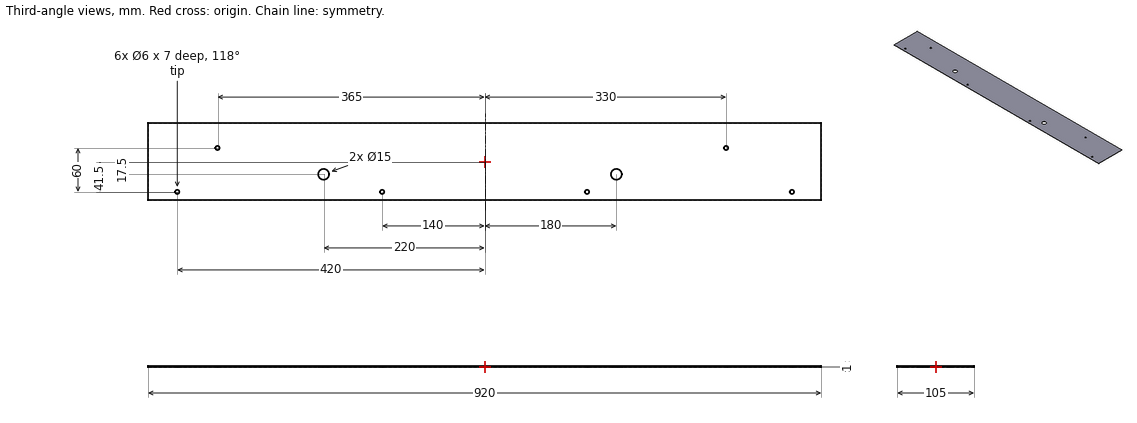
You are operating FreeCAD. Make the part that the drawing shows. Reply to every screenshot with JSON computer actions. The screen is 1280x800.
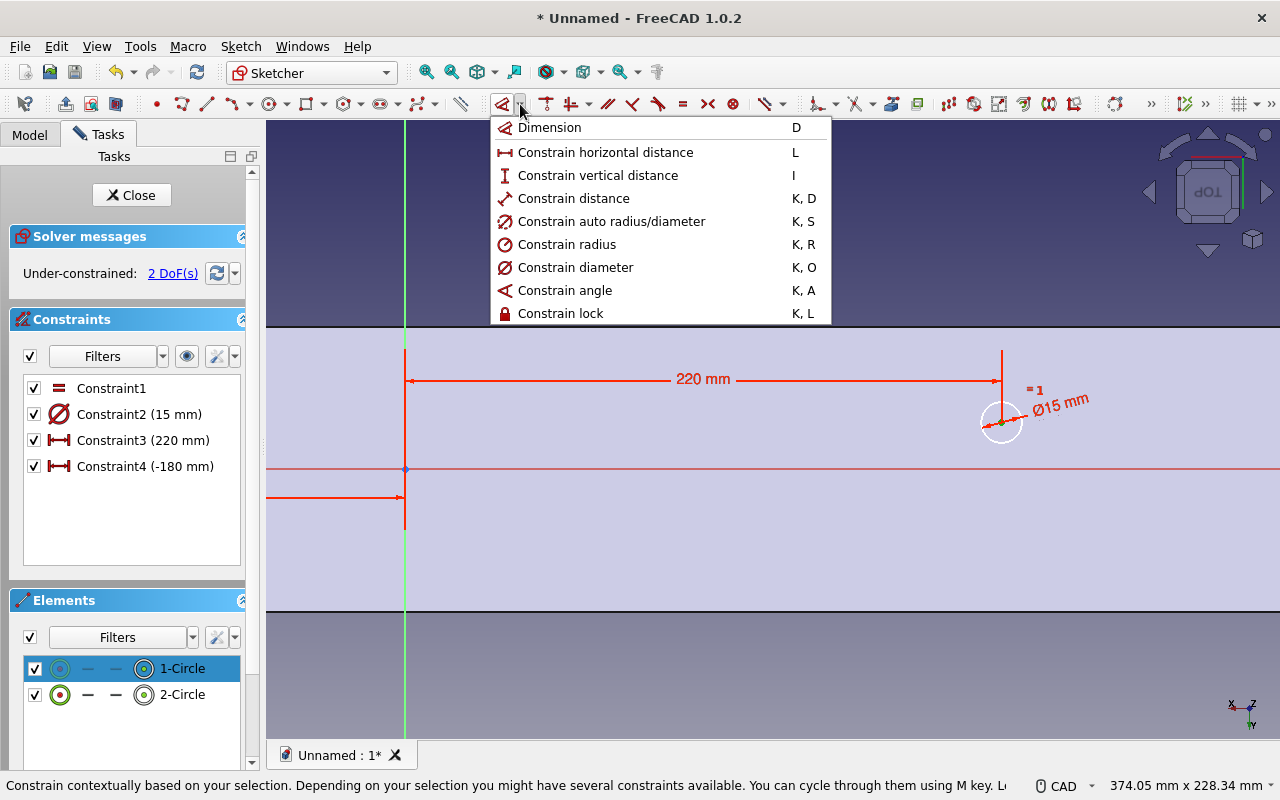
{"action": "left_click", "coordinate": [661, 176]}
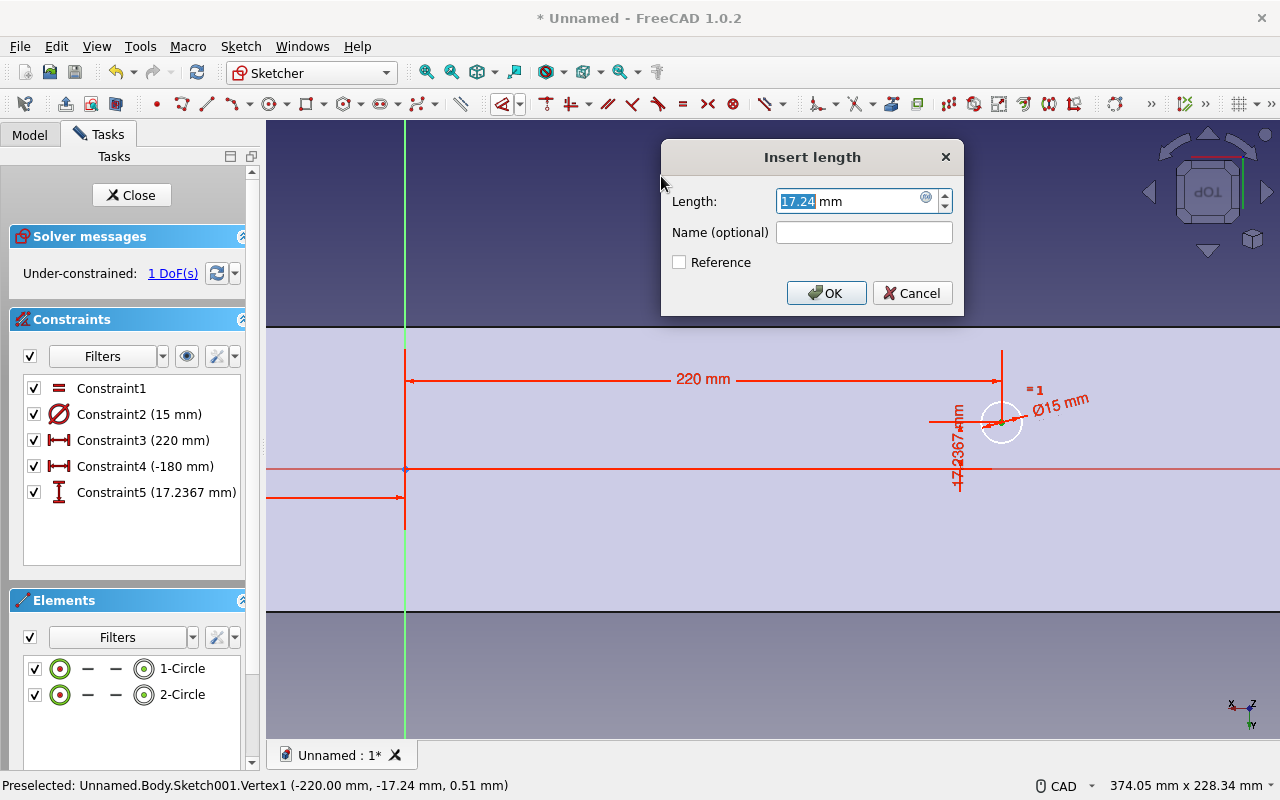
{"action": "type", "text": "17.5"}
{"action": "key", "text": "Return"}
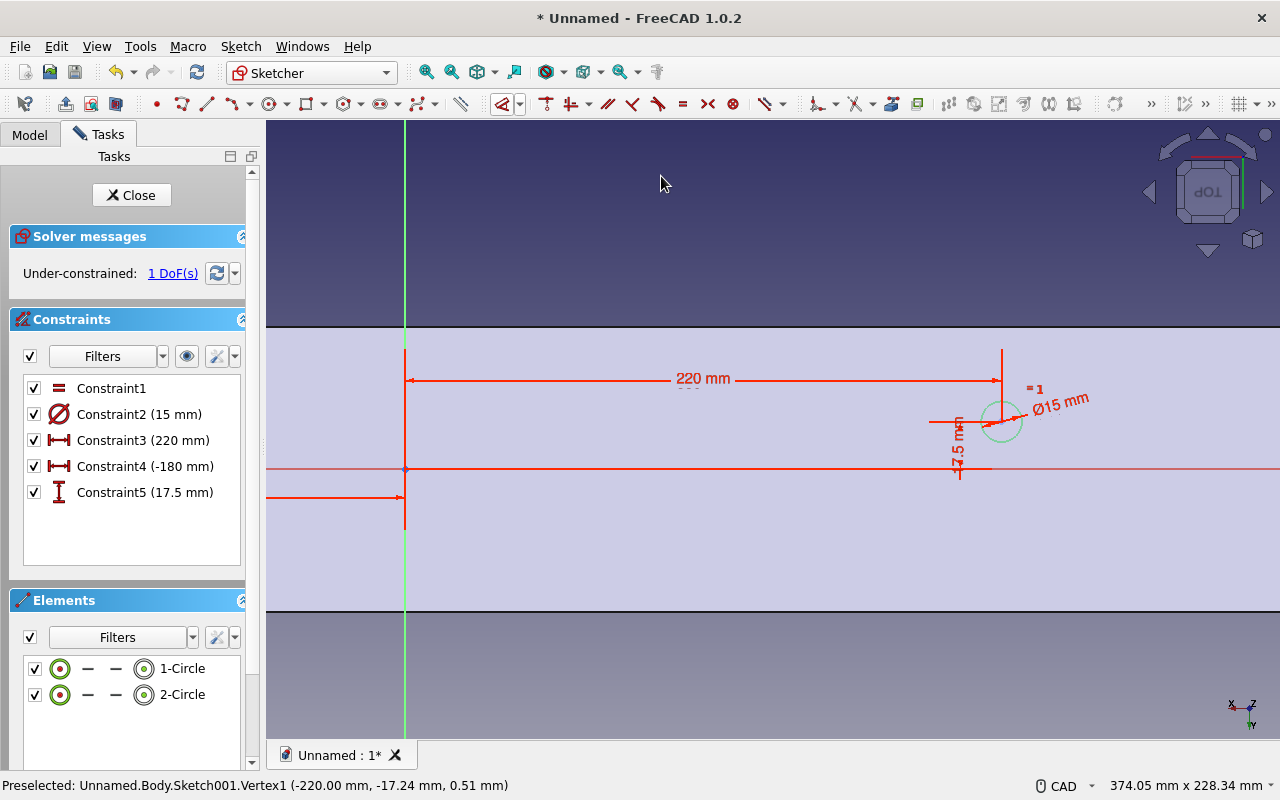
{"action": "scroll", "coordinate": [1003, 422], "scroll_direction": "down", "scroll_amount": 3}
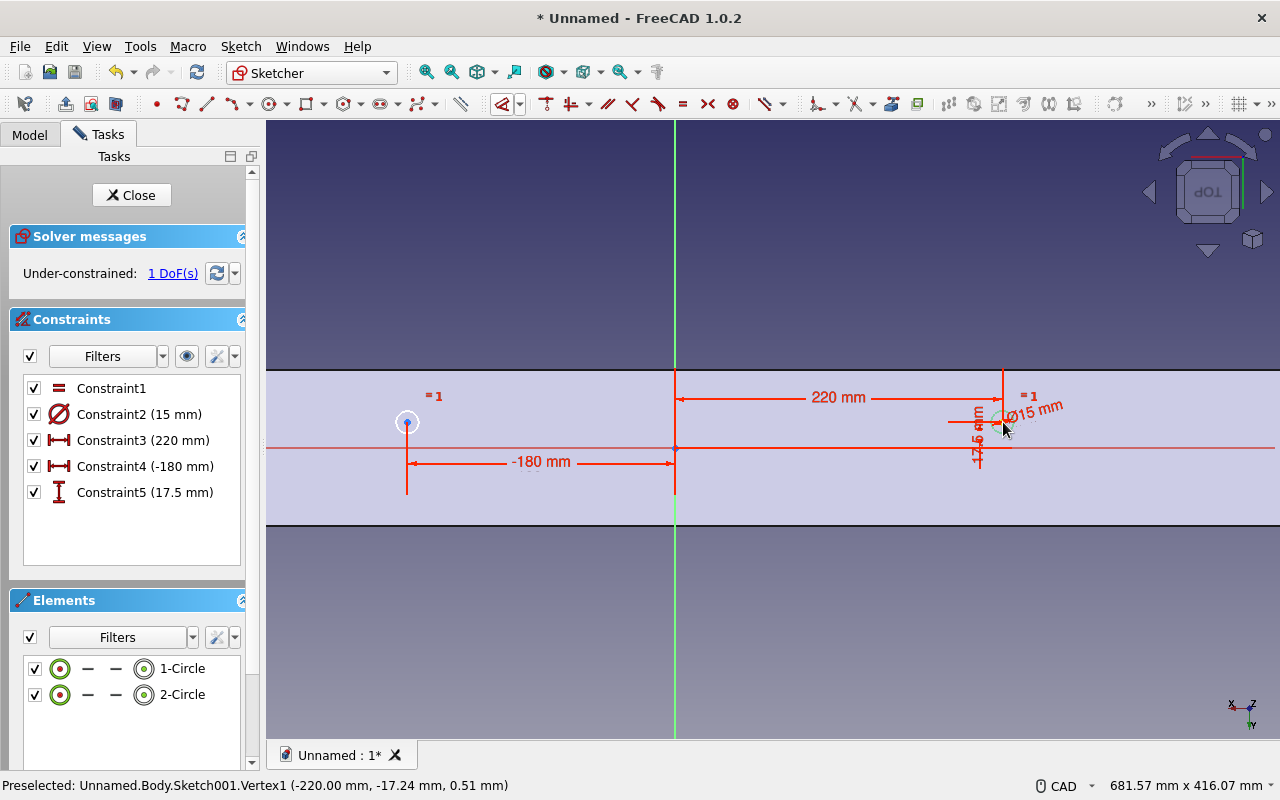
{"action": "scroll", "coordinate": [407, 422], "scroll_direction": "up", "scroll_amount": 3}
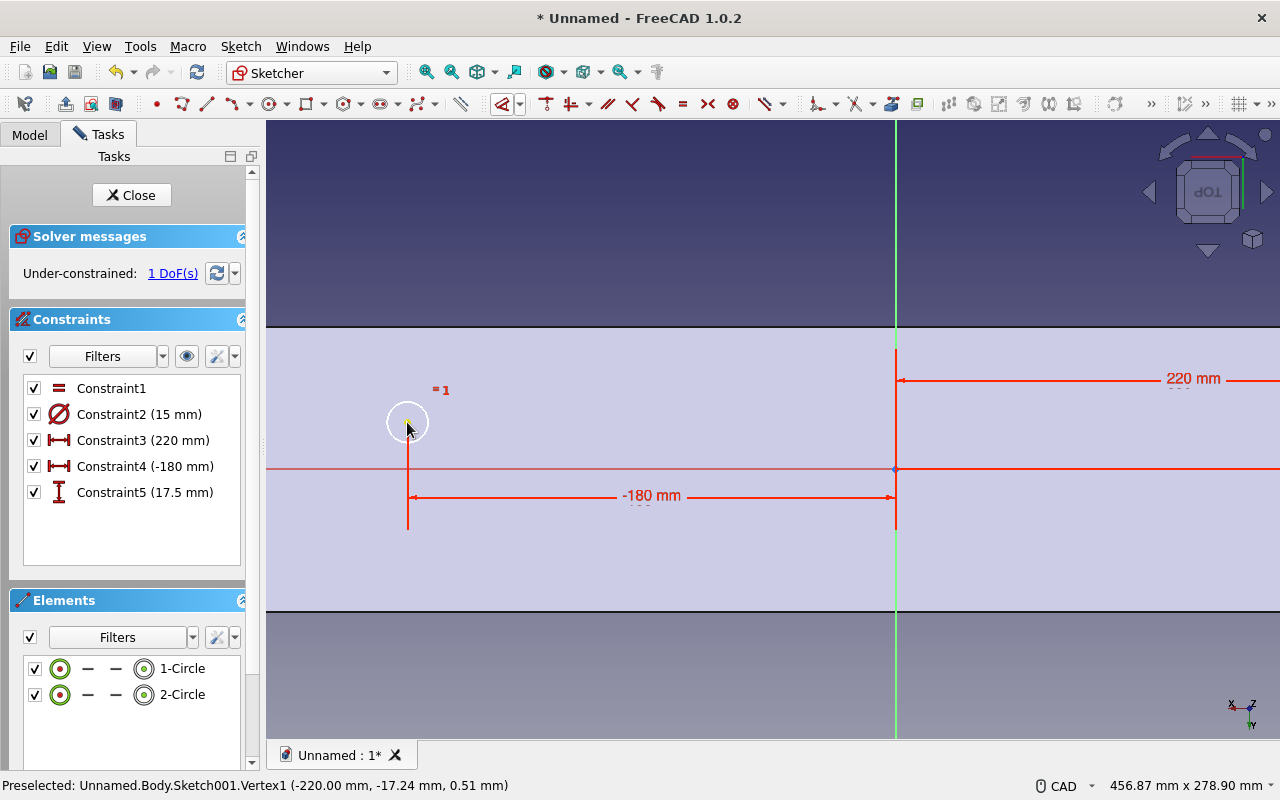
{"action": "left_click", "coordinate": [408, 422]}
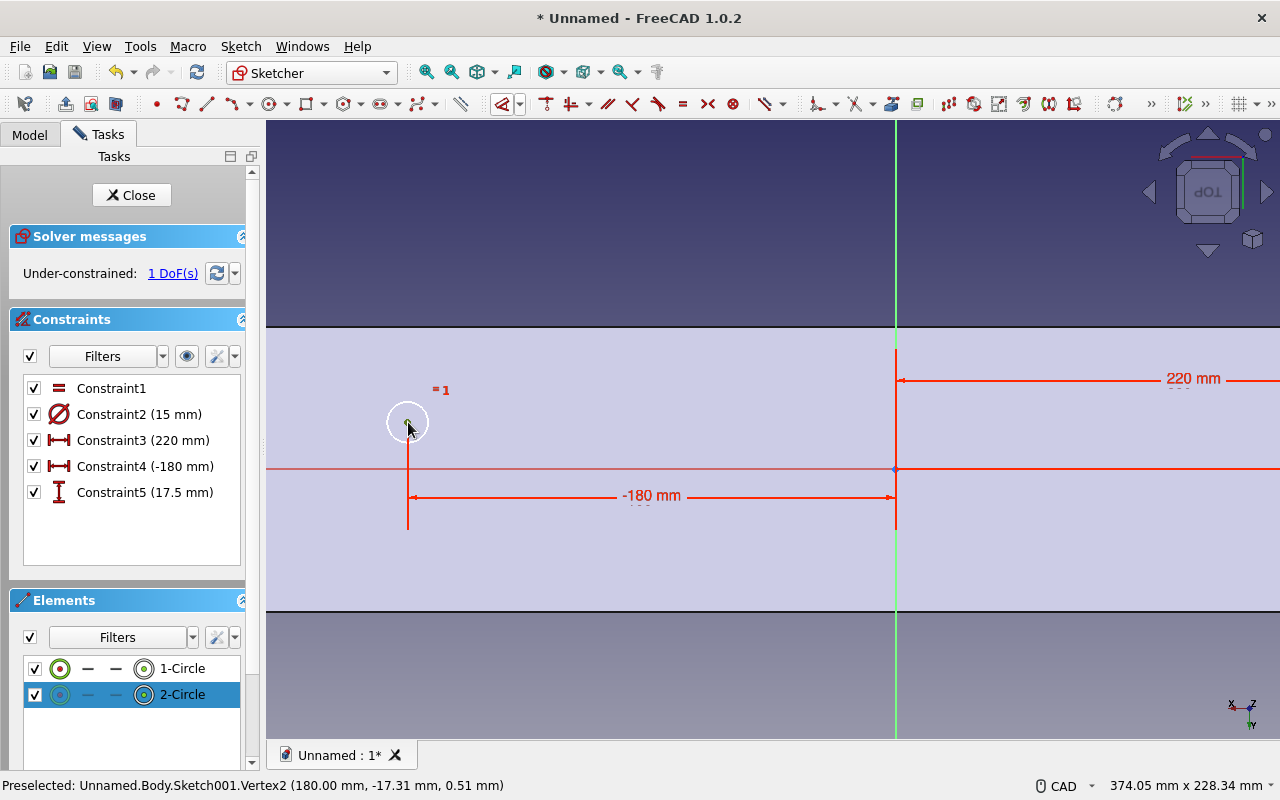
{"action": "left_click", "coordinate": [520, 104]}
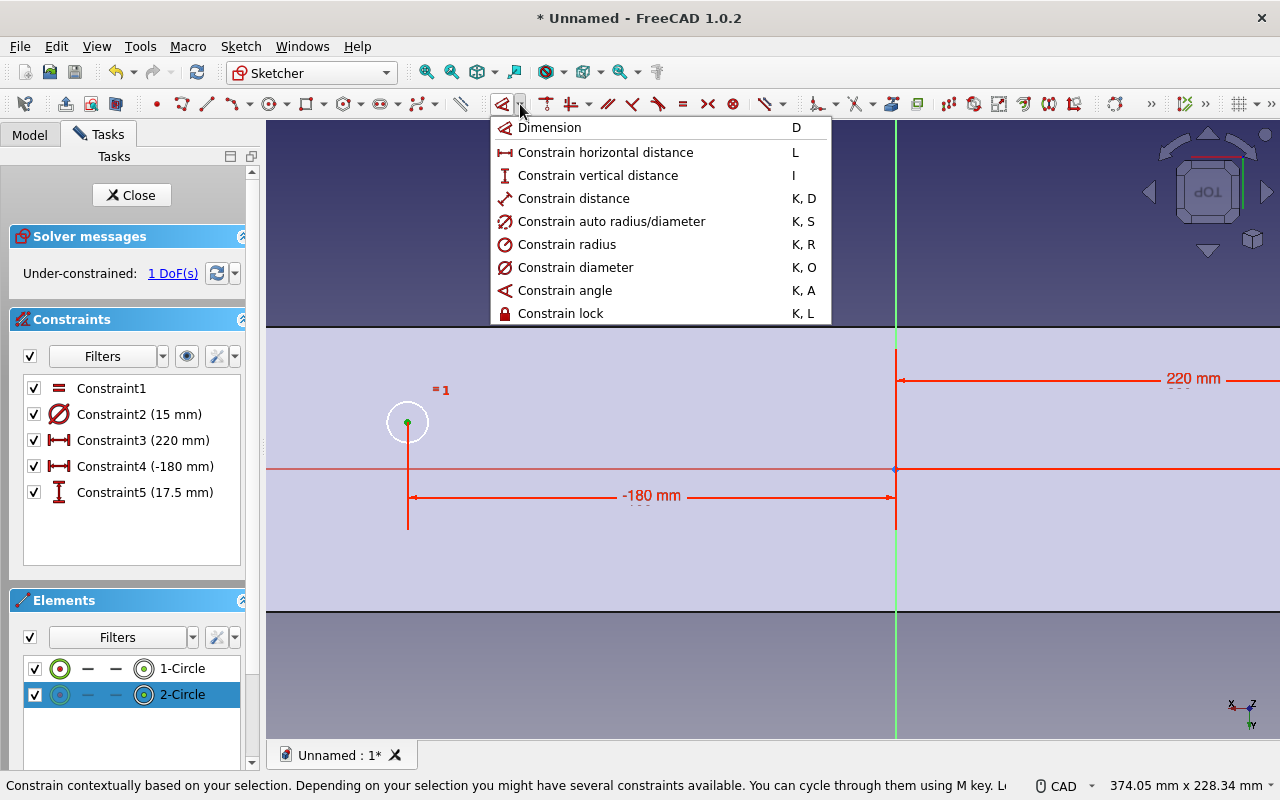
{"action": "left_click", "coordinate": [661, 176]}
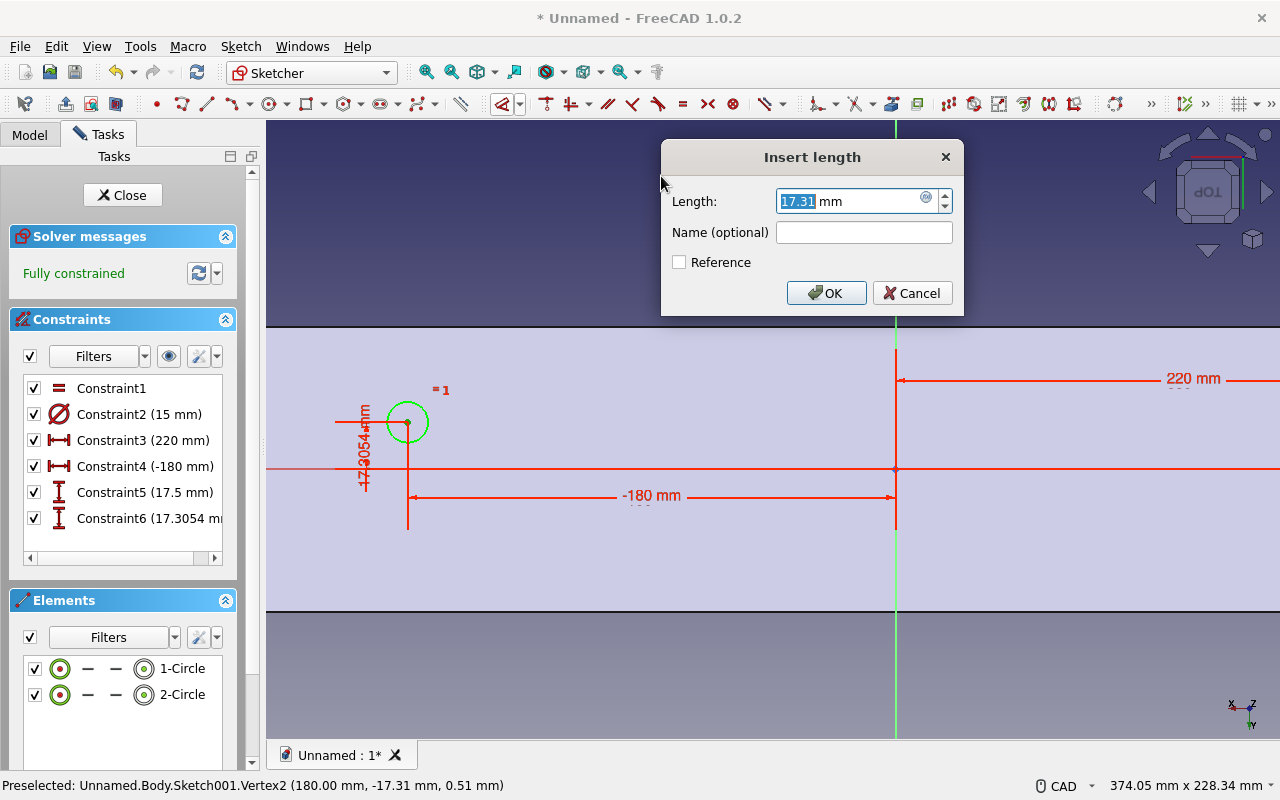
{"action": "type", "text": "17.5"}
{"action": "key", "text": "Return"}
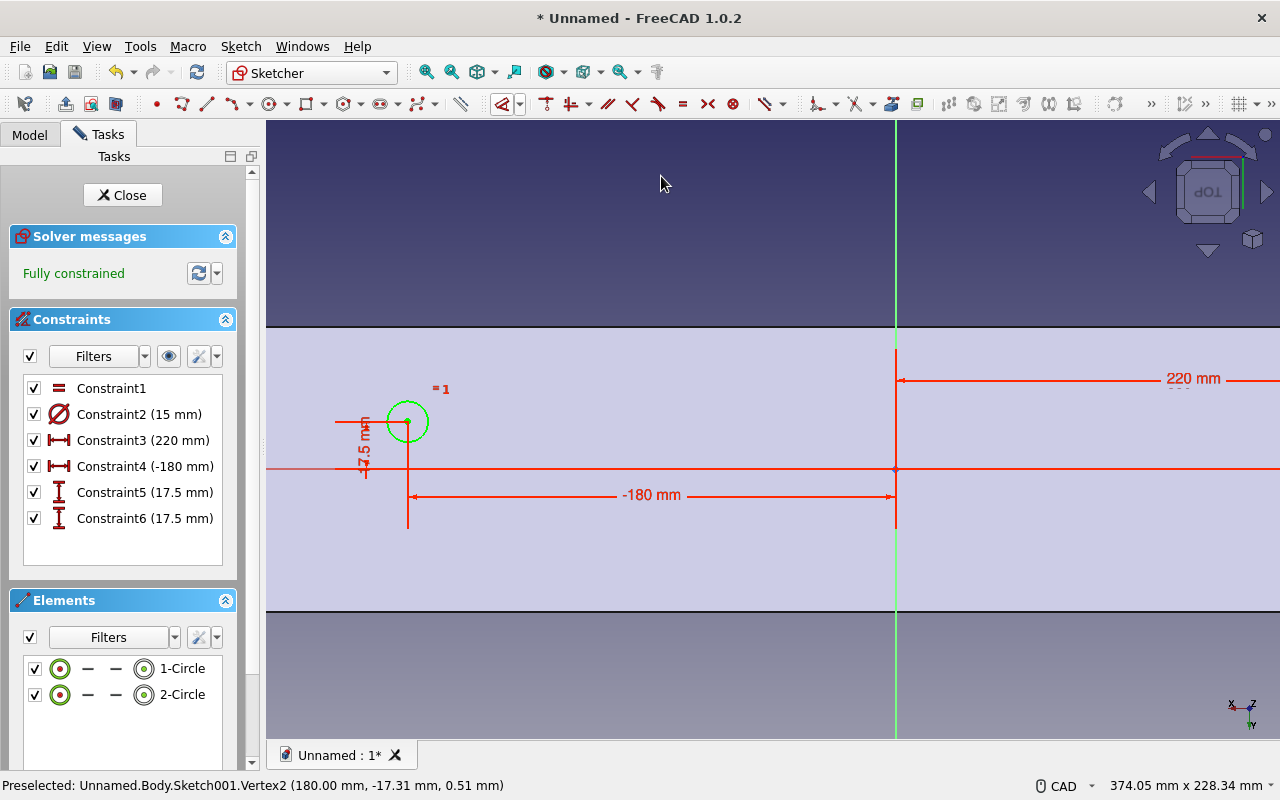
{"action": "left_click", "coordinate": [123, 195]}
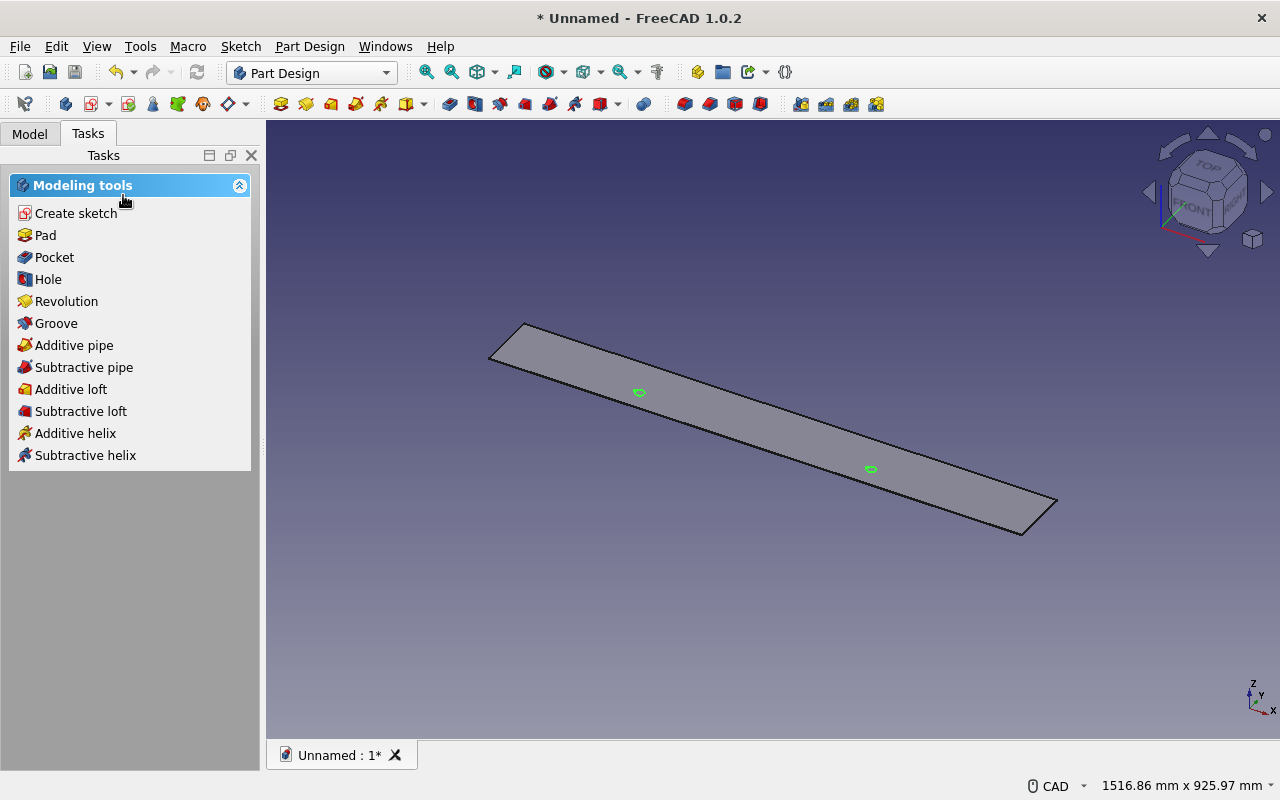
{"action": "left_click", "coordinate": [450, 104]}